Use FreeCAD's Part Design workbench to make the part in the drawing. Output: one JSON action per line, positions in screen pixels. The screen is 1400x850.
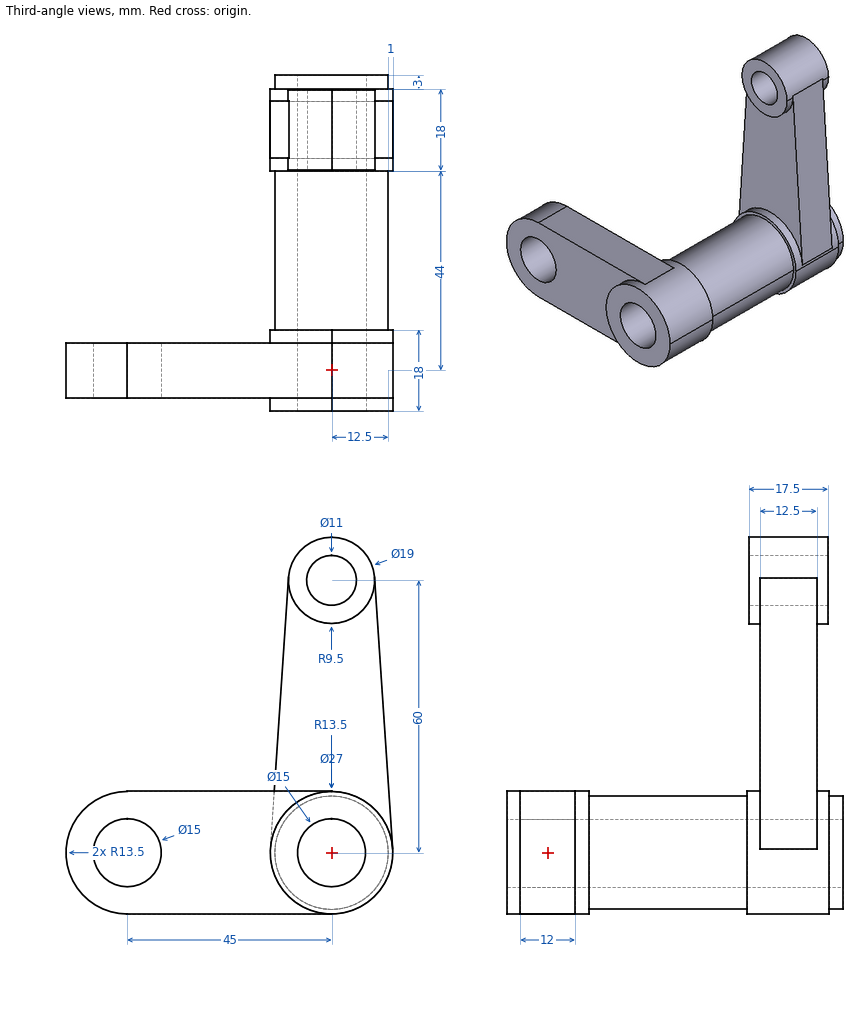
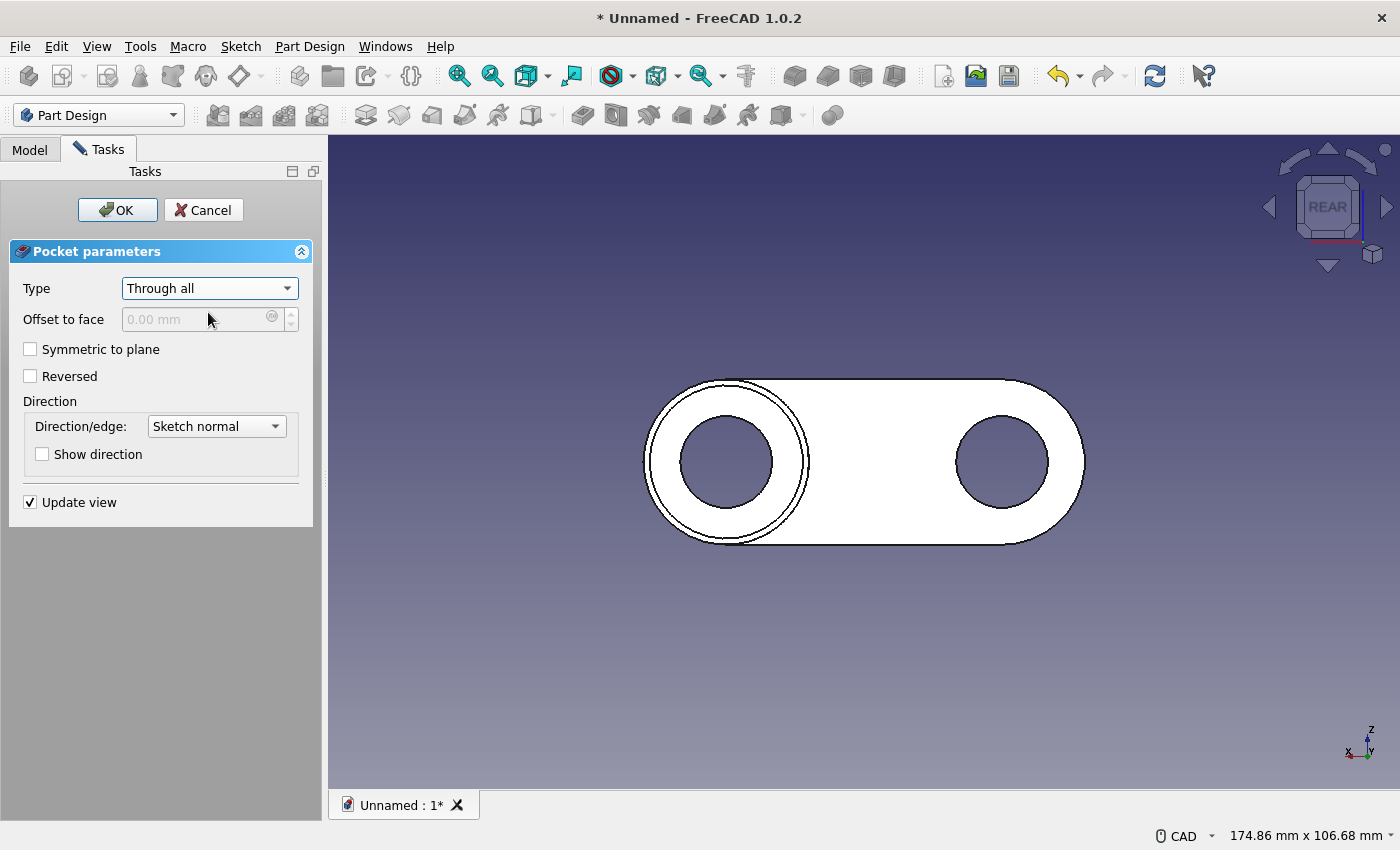
{"action": "left_click", "coordinate": [118, 210]}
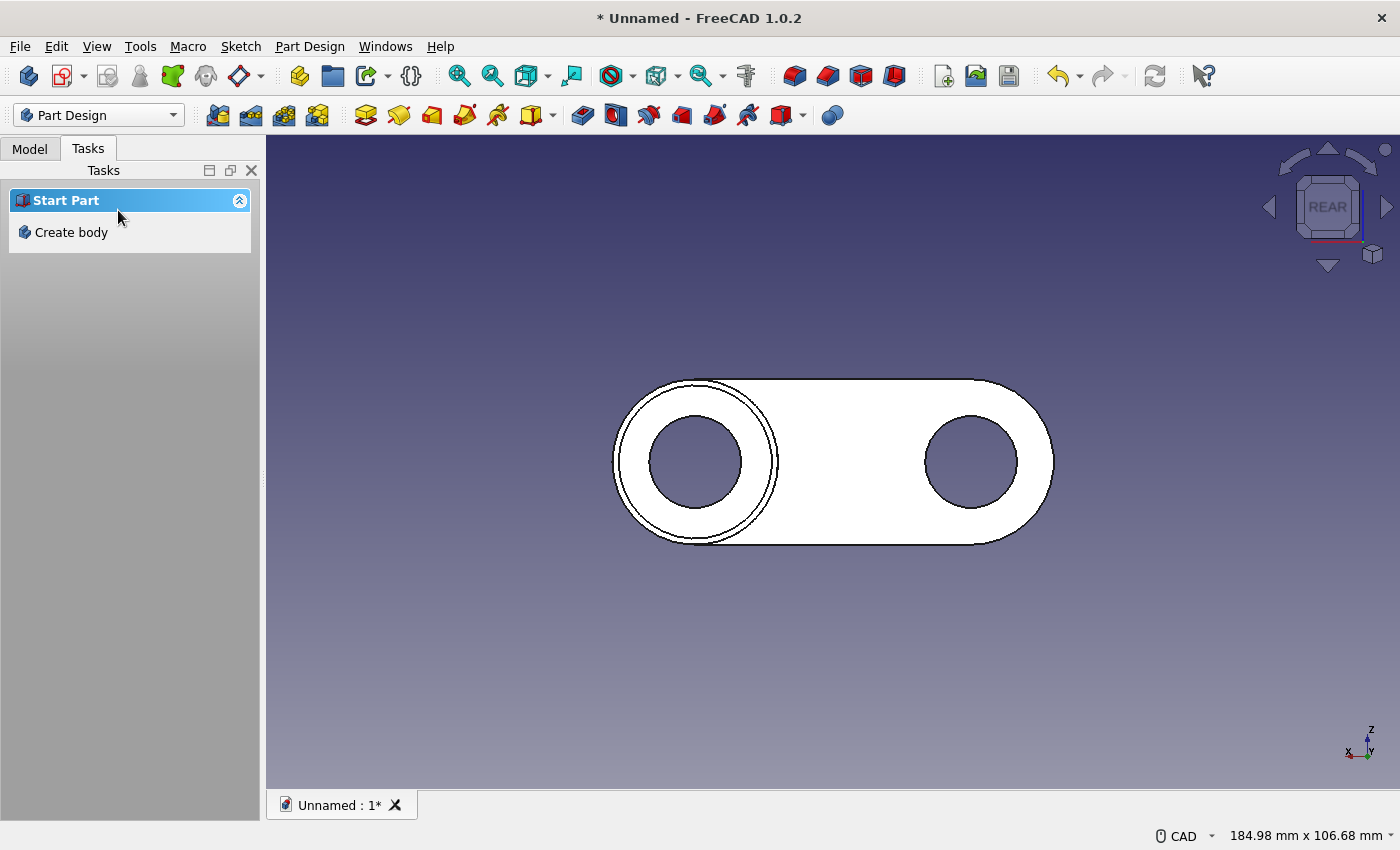
{"action": "key", "text": "v f"}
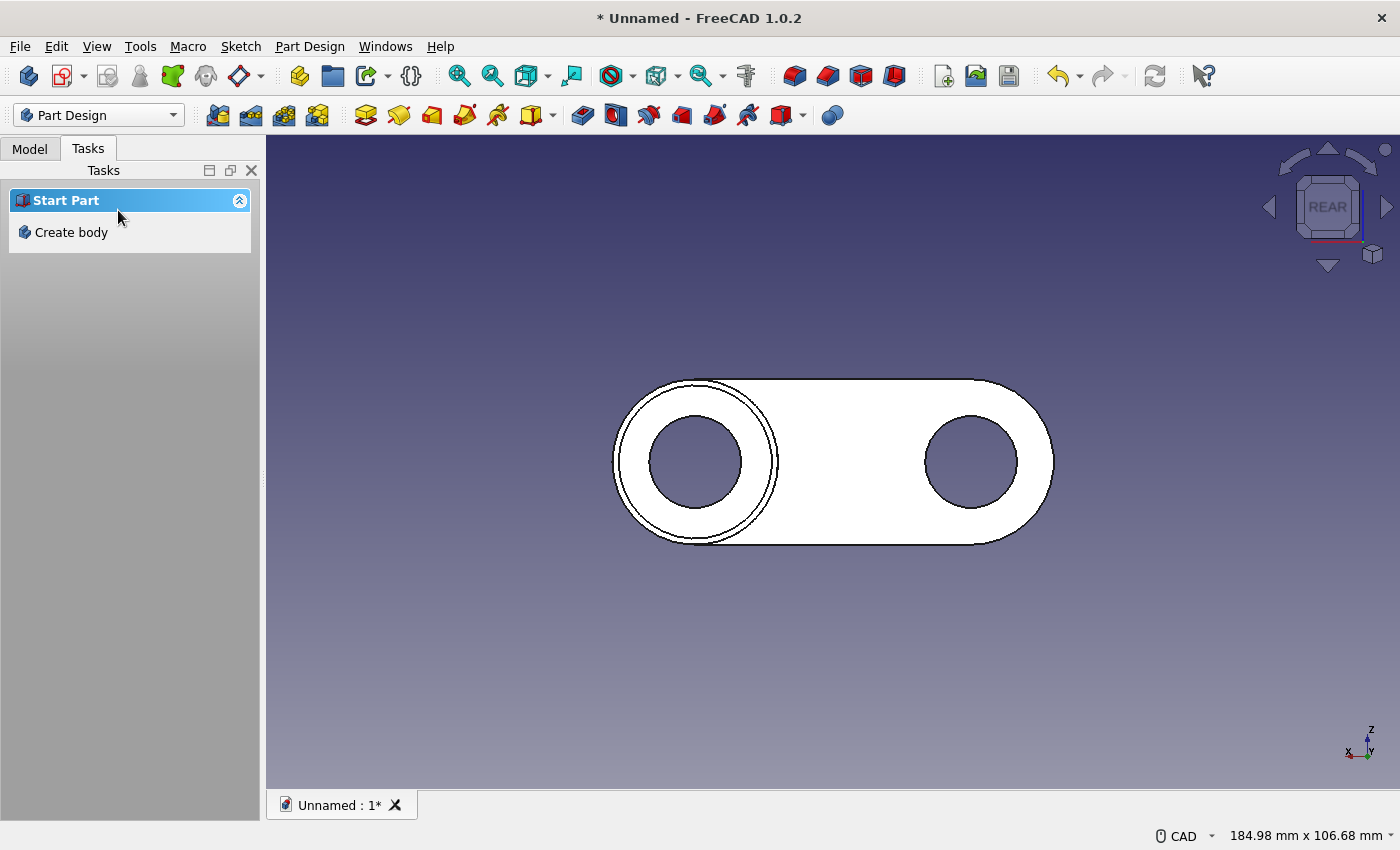
{"action": "left_click", "coordinate": [29, 76]}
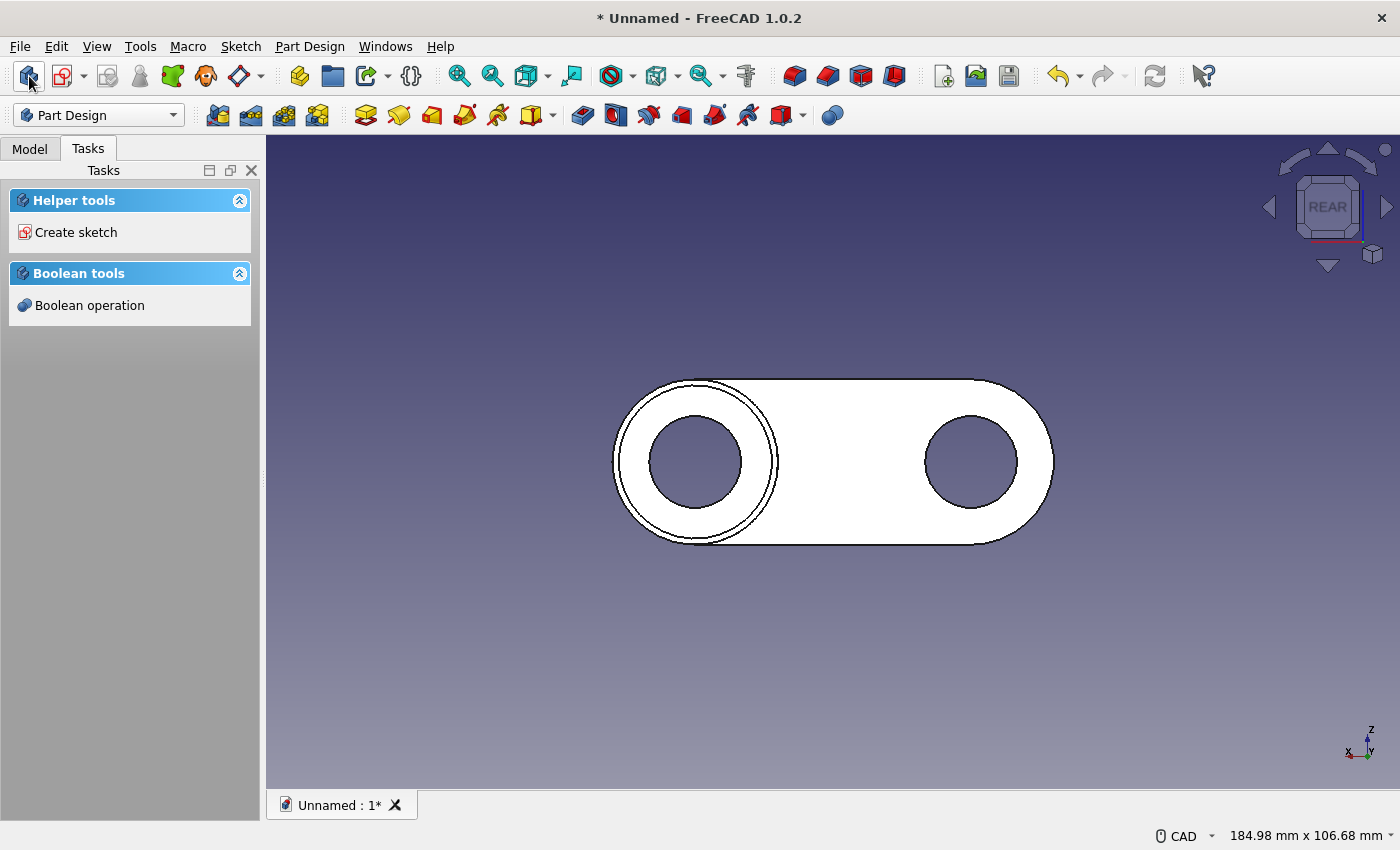
{"action": "left_click", "coordinate": [30, 148]}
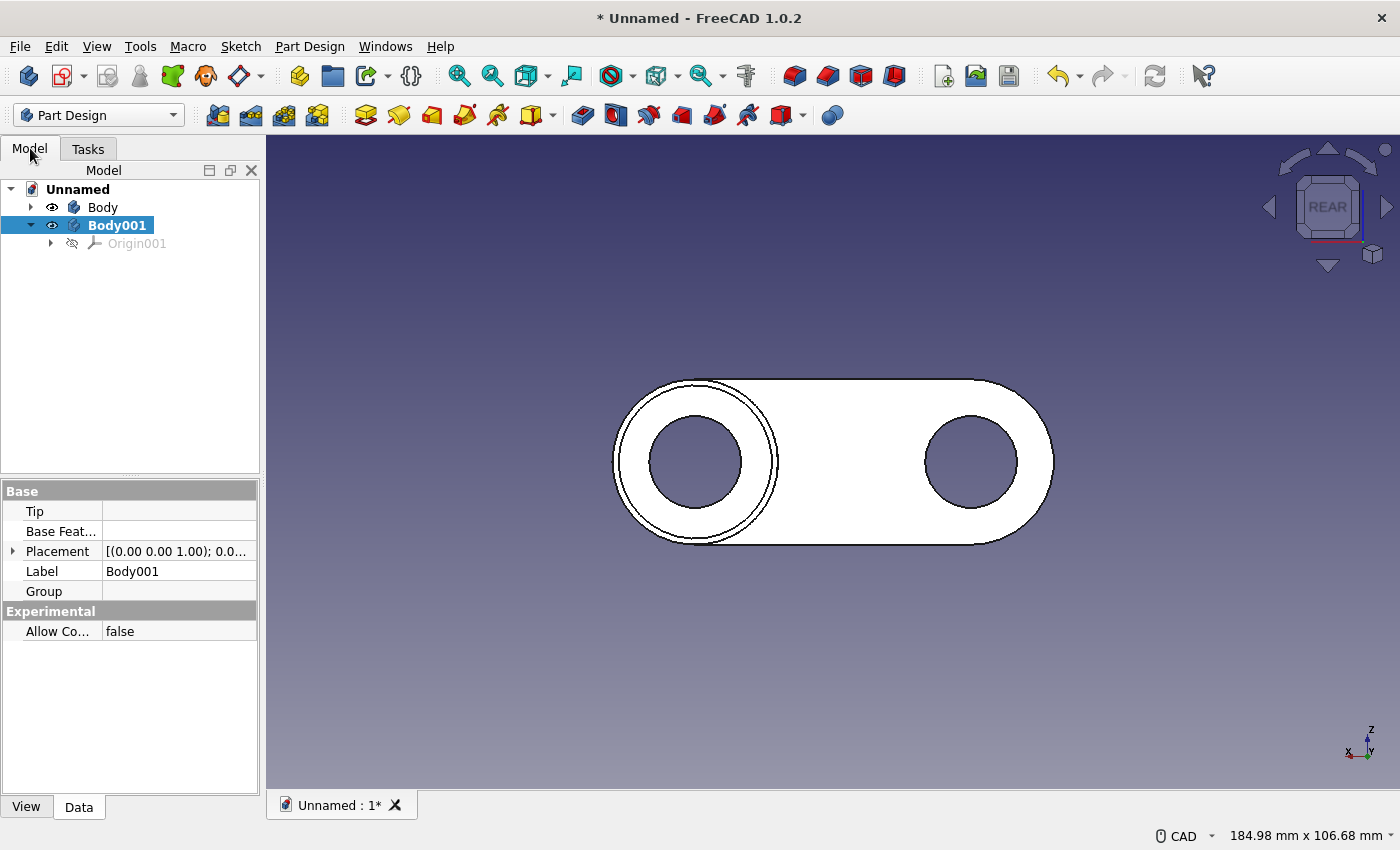
{"action": "left_click", "coordinate": [51, 243]}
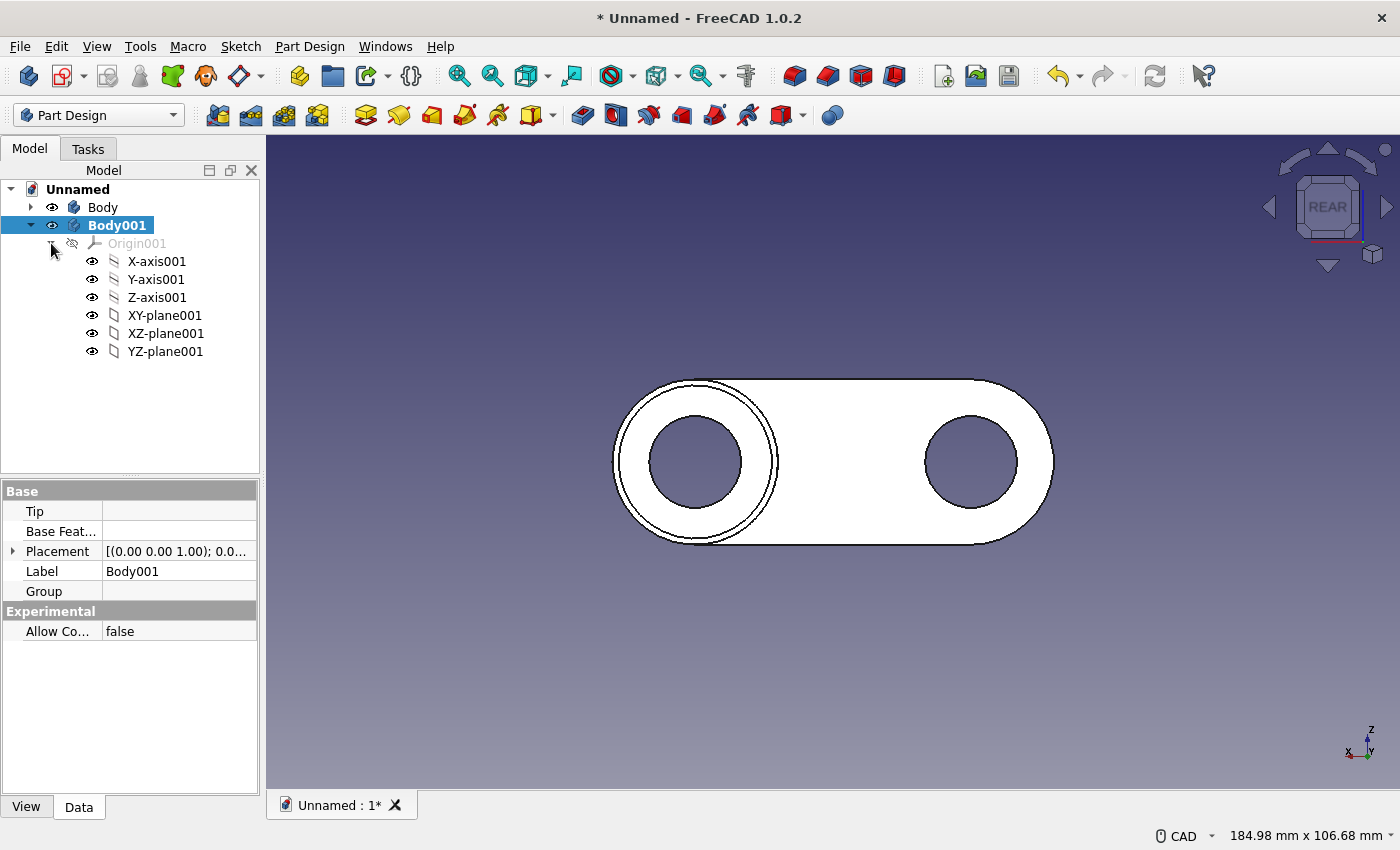
{"action": "left_click", "coordinate": [137, 333]}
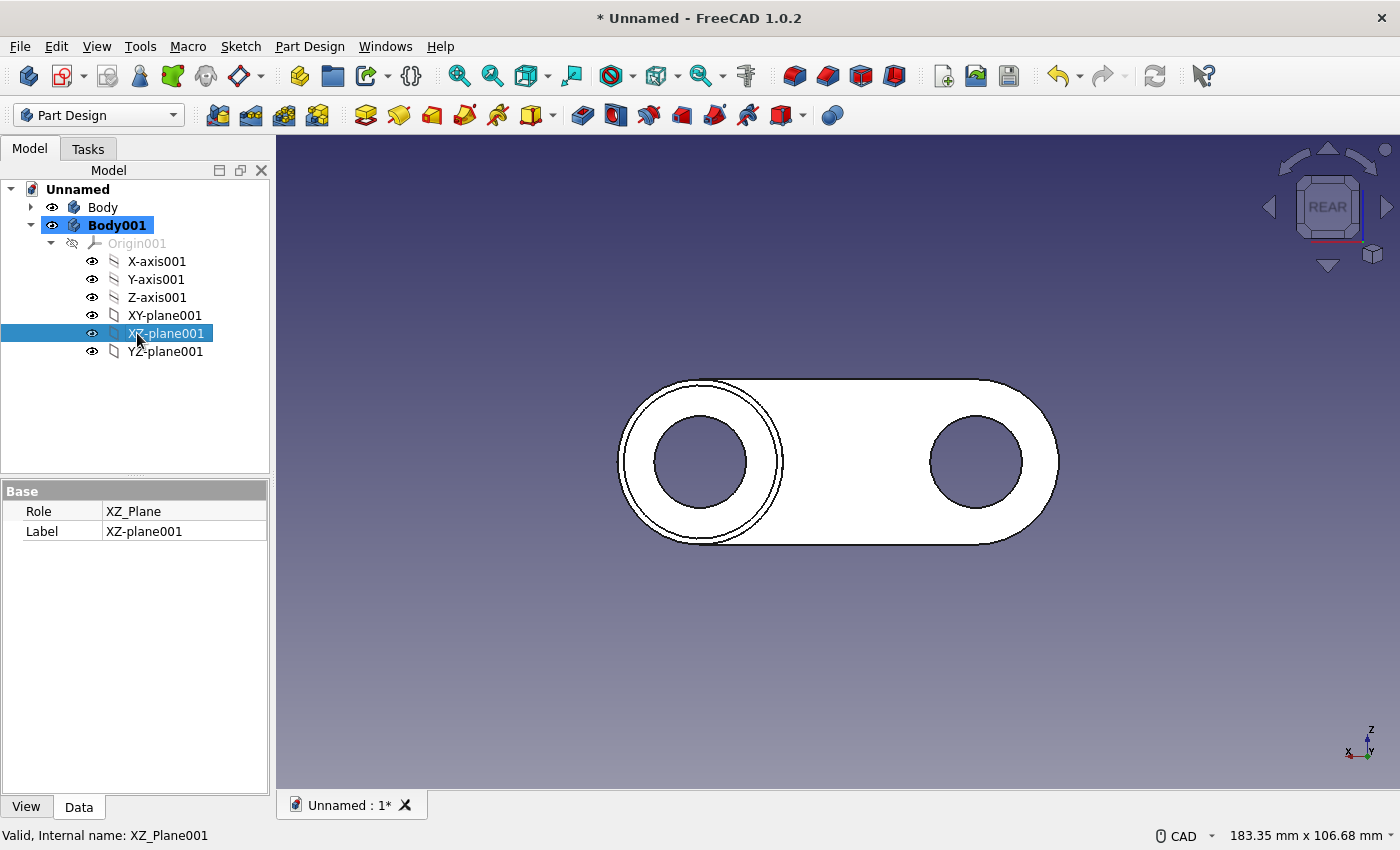
{"action": "left_click", "coordinate": [238, 76]}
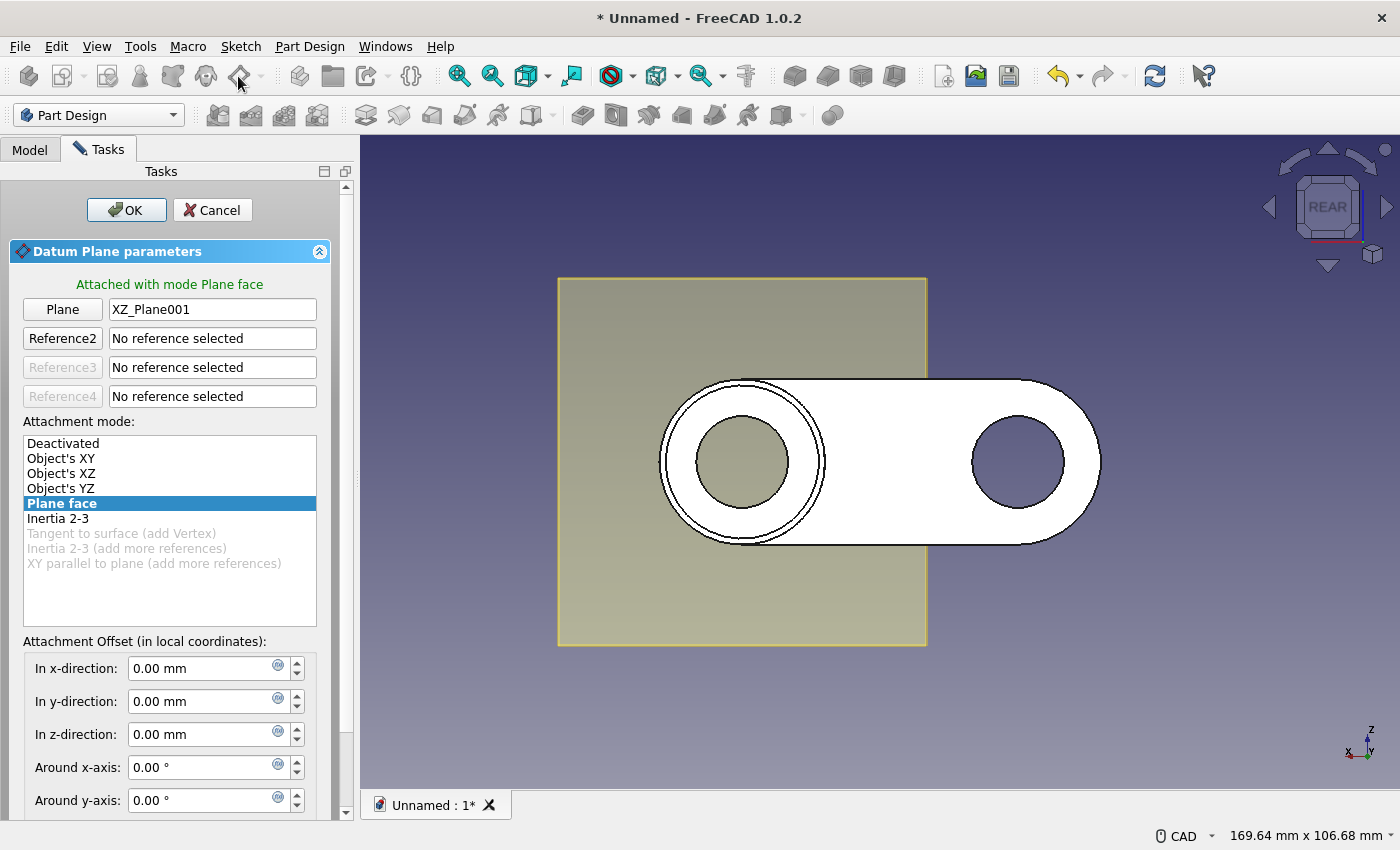
{"action": "triple_click", "coordinate": [210, 734]}